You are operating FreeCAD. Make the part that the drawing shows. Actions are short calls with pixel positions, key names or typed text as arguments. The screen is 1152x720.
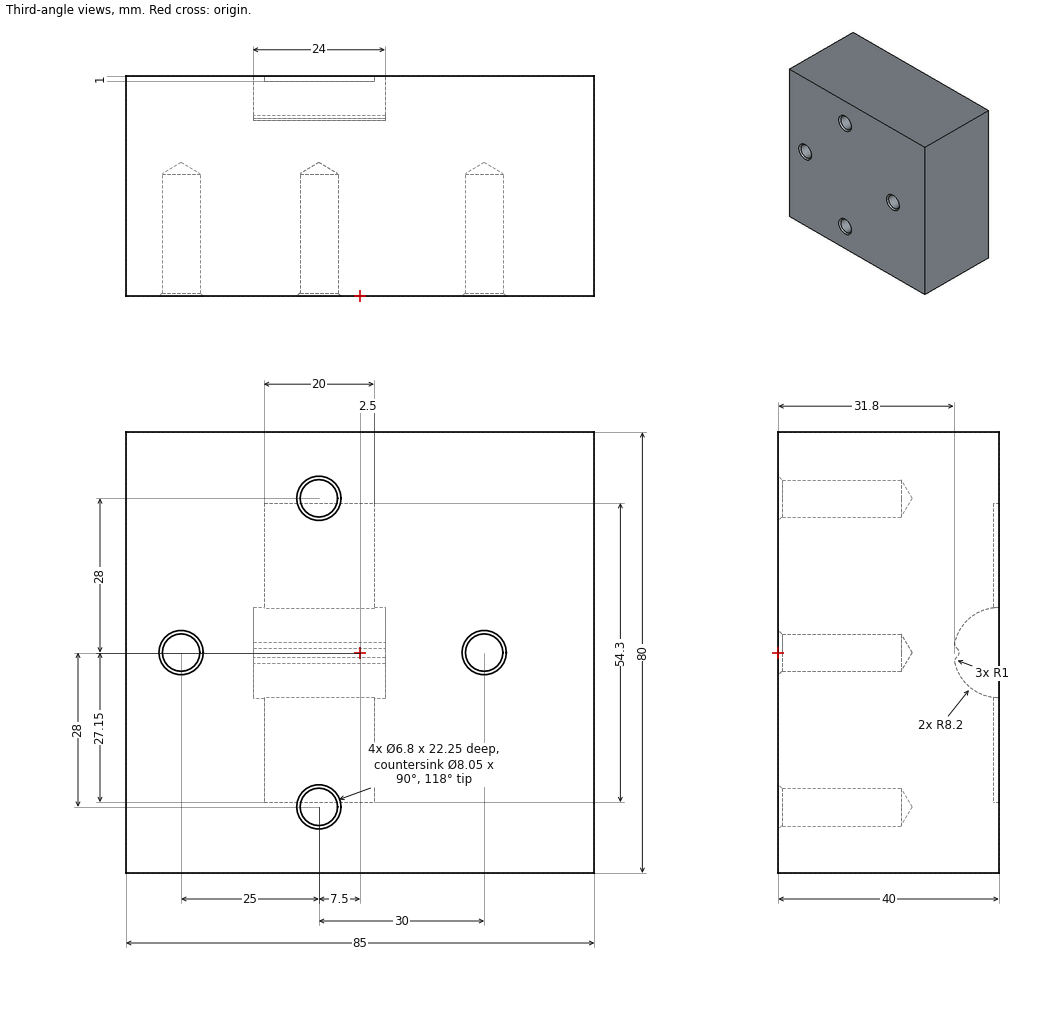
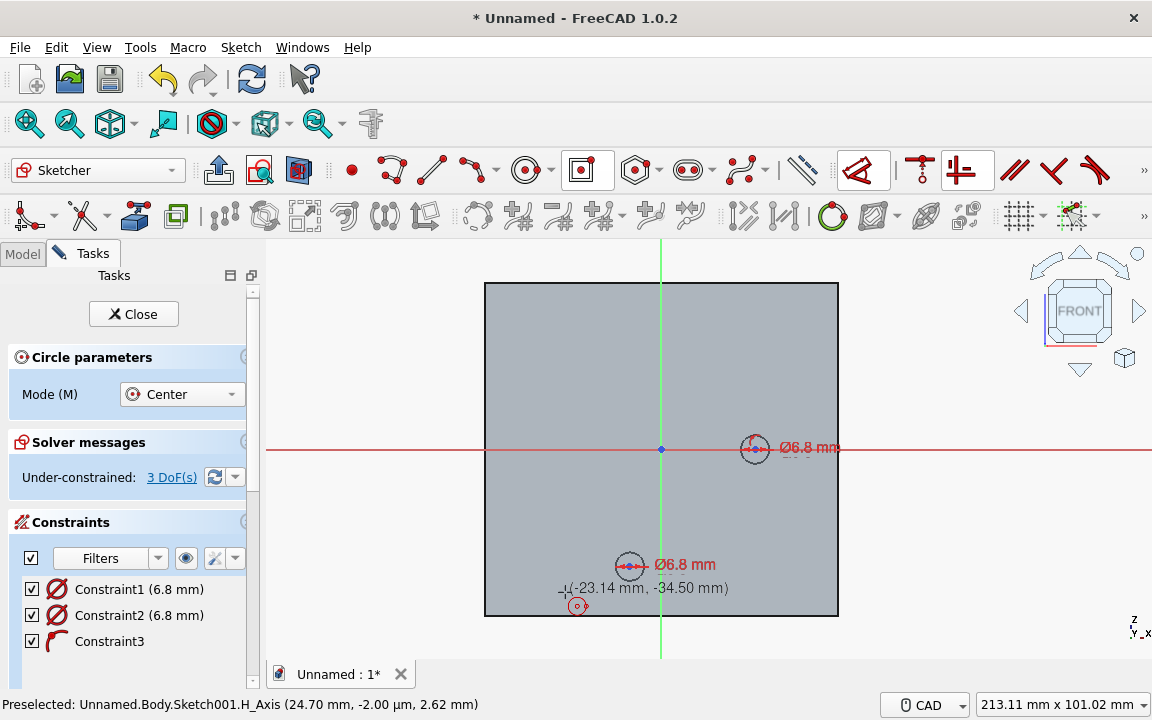
scroll(630, 333, up, 3)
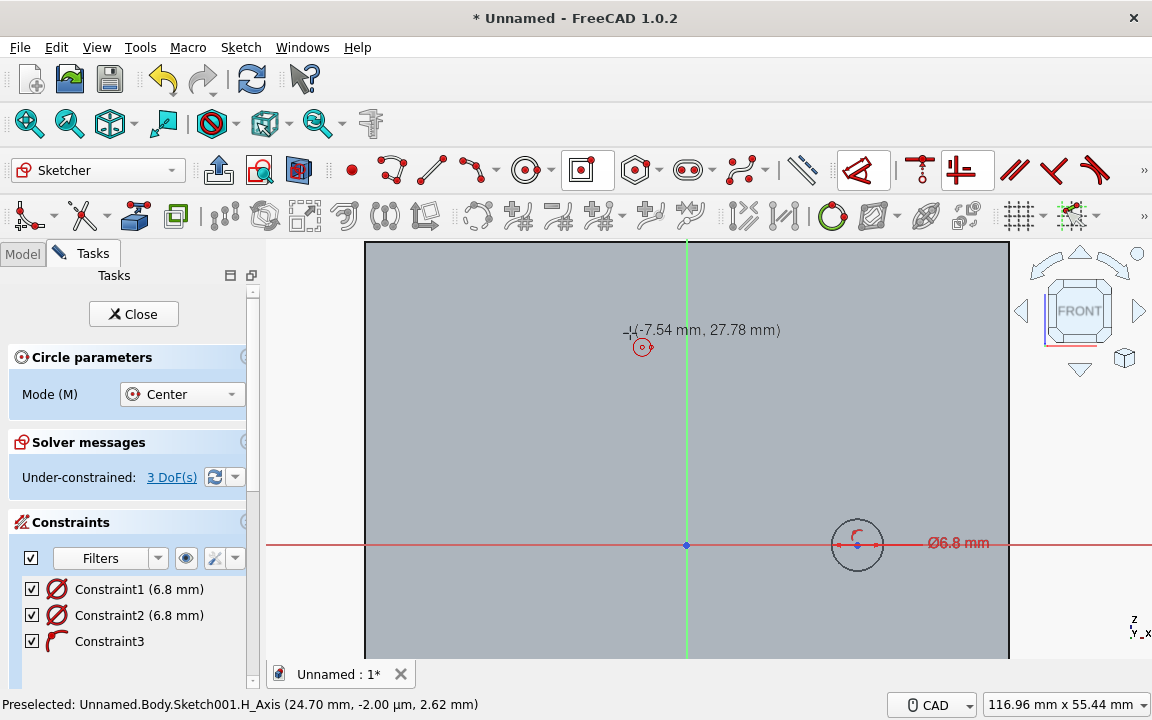
click(630, 333)
move(648, 315)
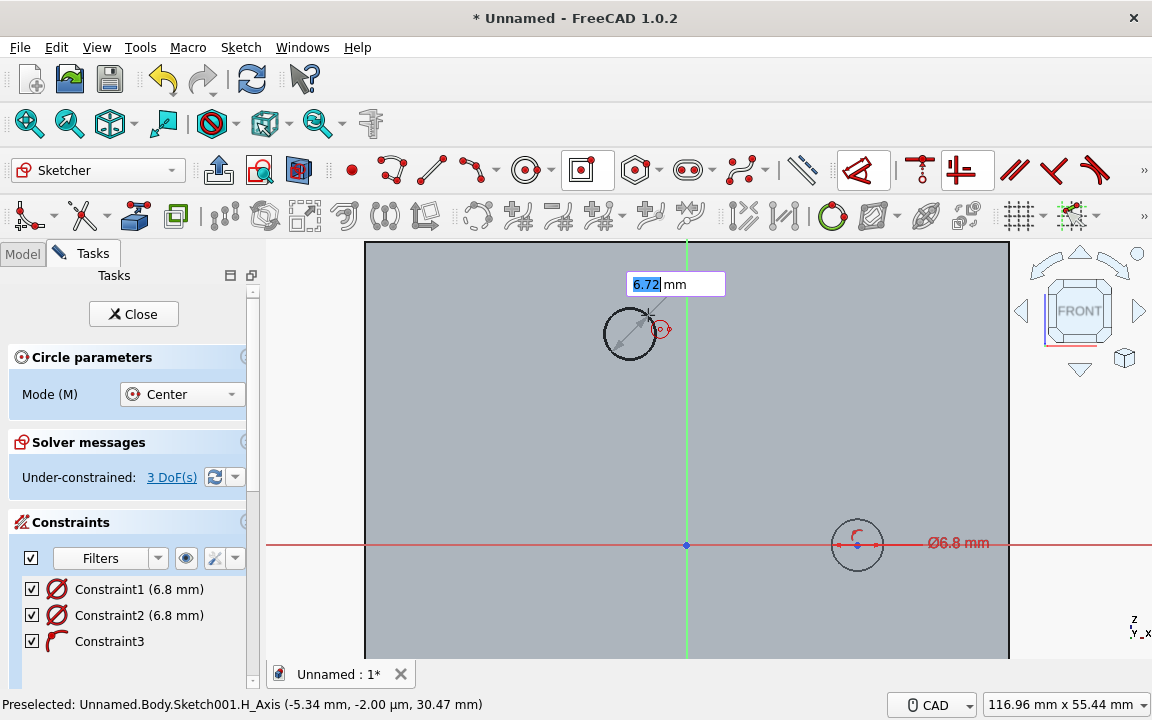
text(6.8)
key(Return)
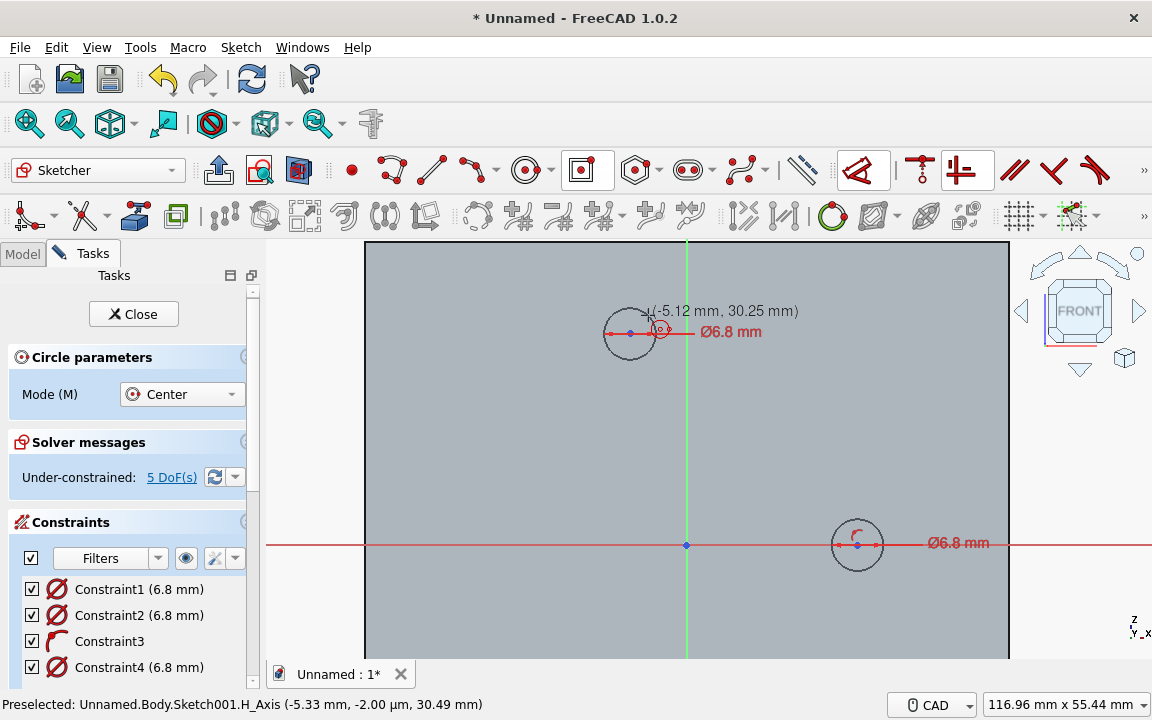
click(441, 545)
move(459, 527)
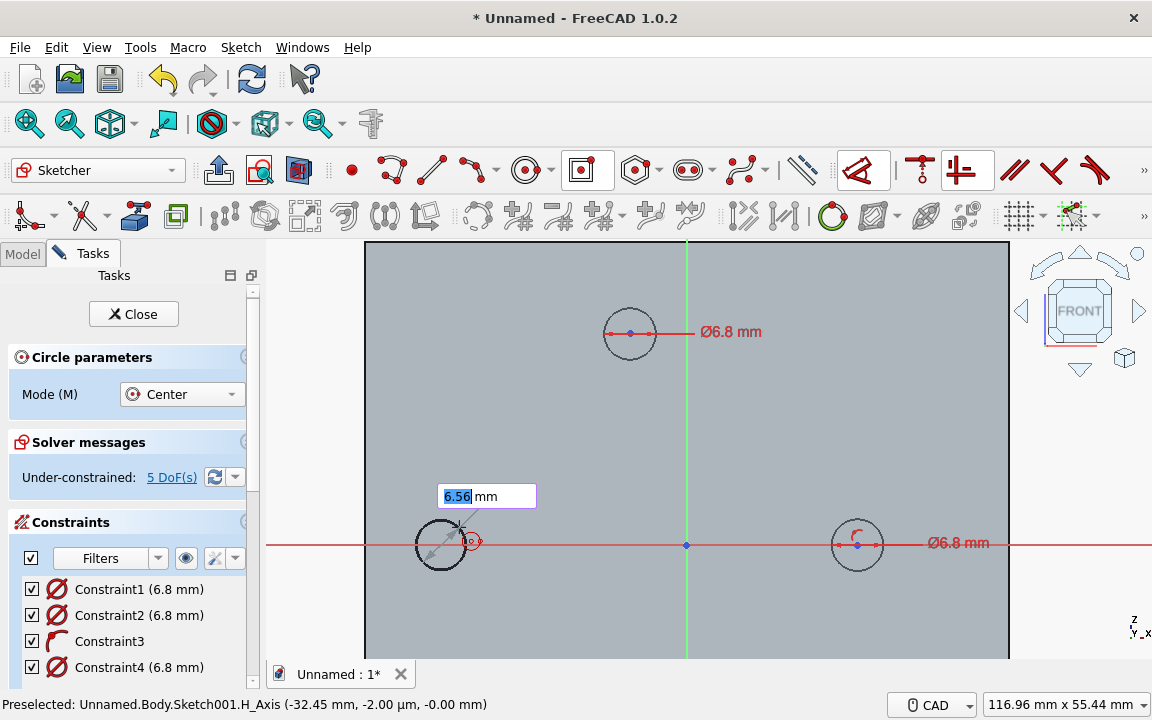
text(6.8)
key(Return)
key(Escape)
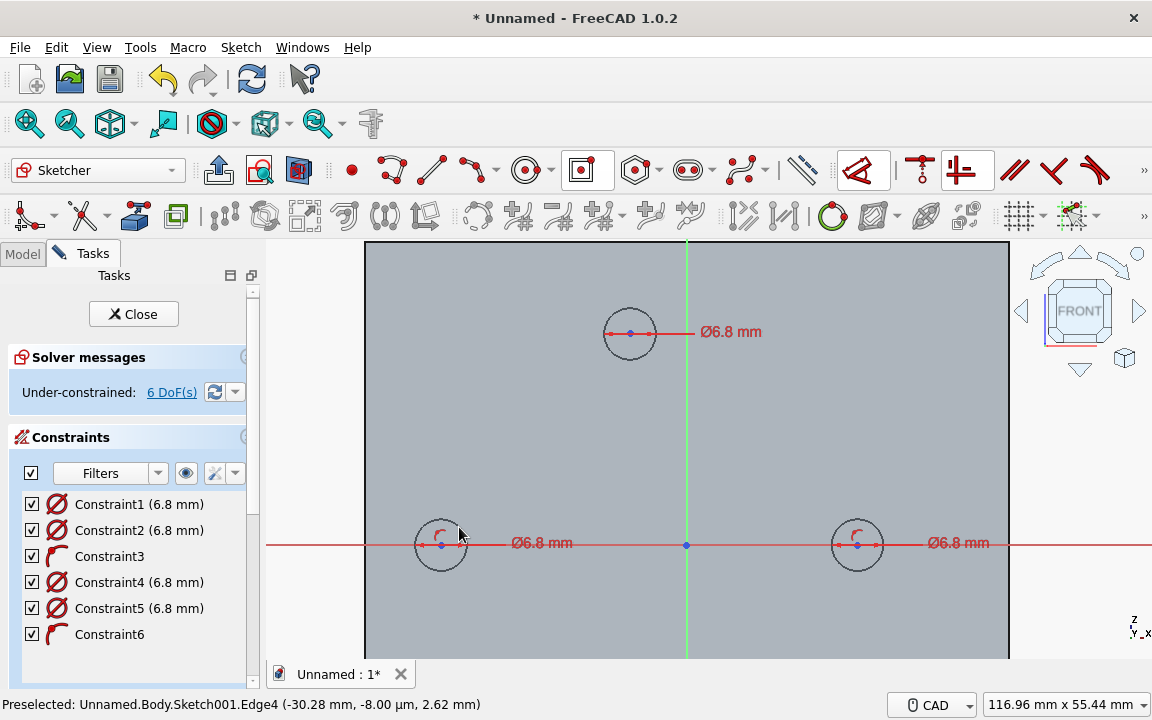
scroll(630, 332, down, 3)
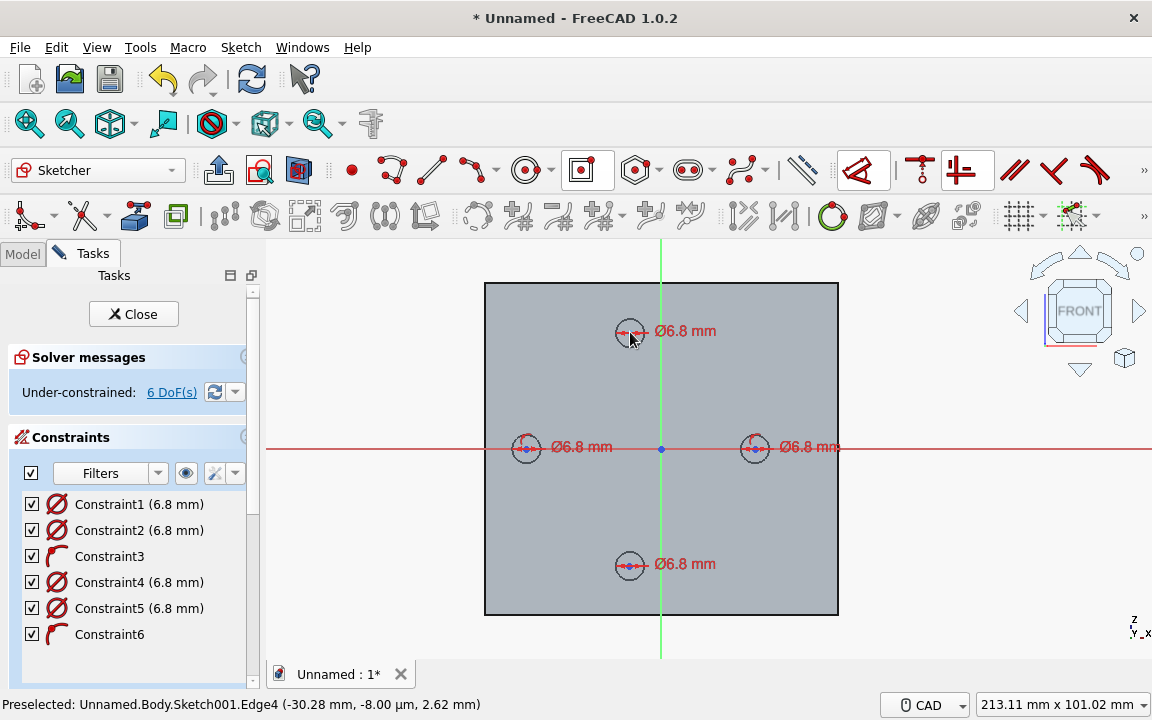
click(630, 566)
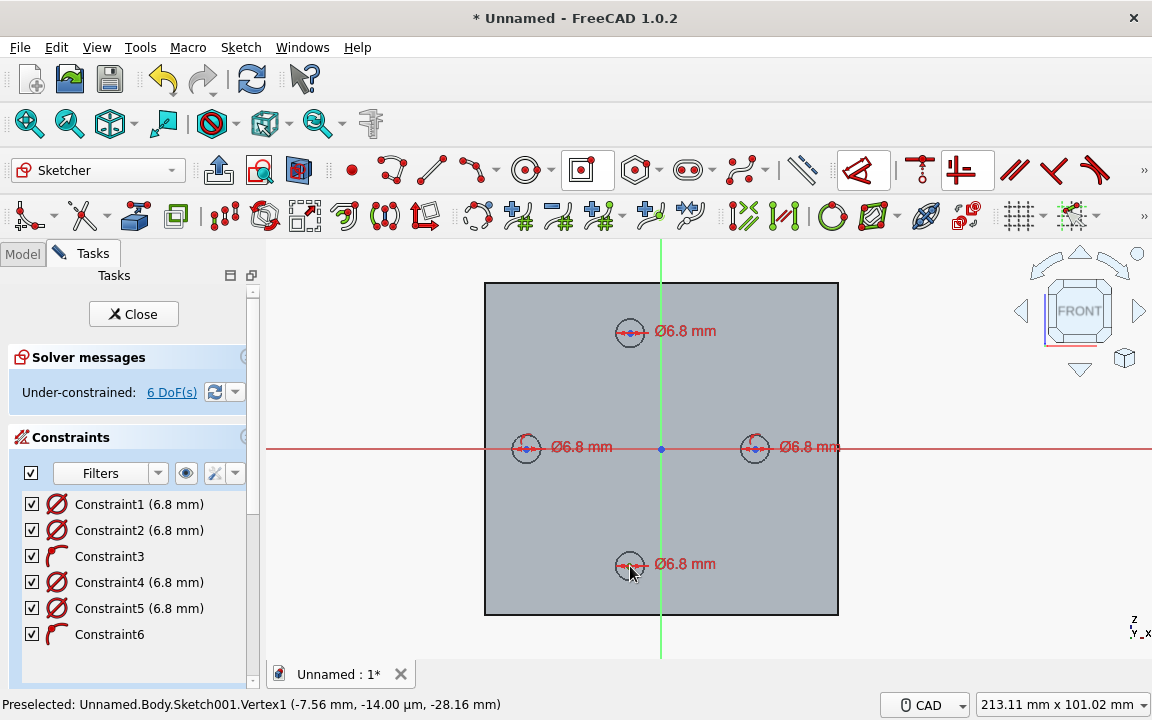
click(630, 333)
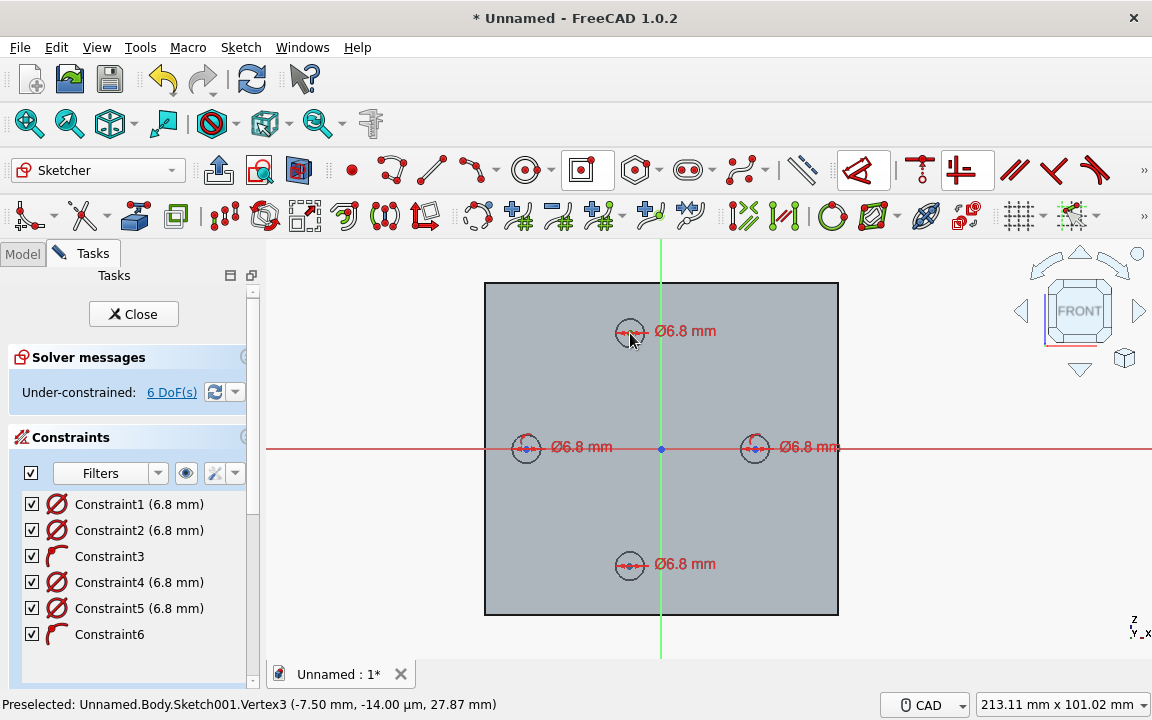
key(v)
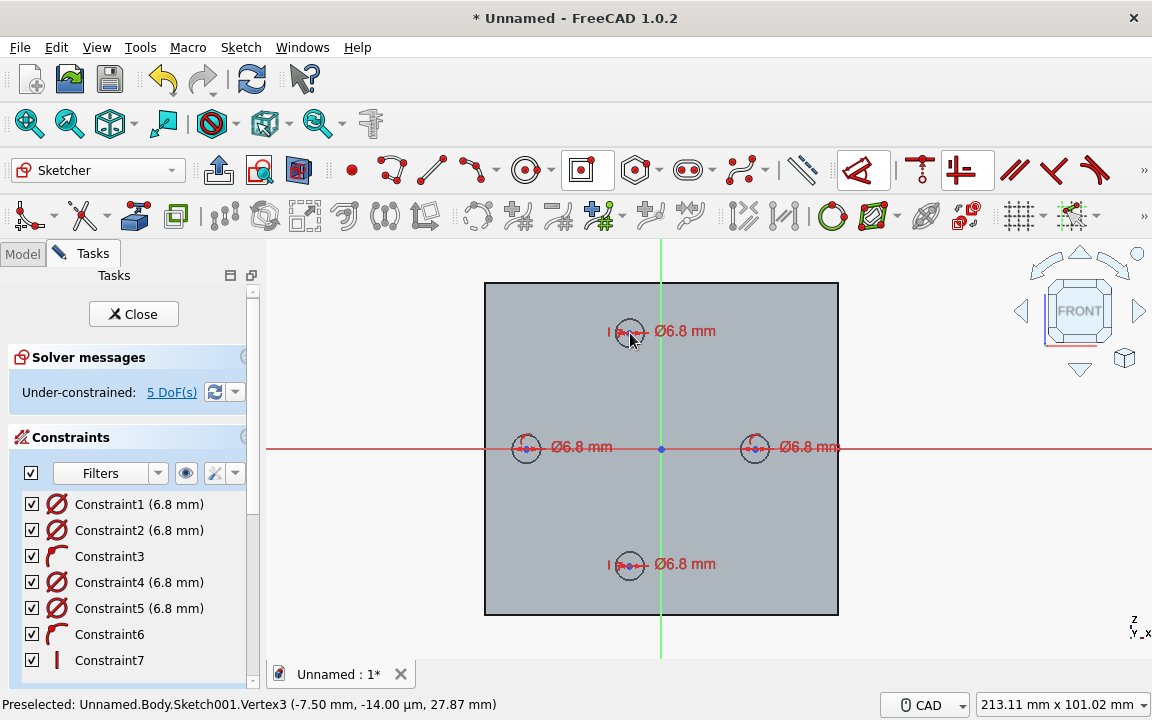
click(858, 170)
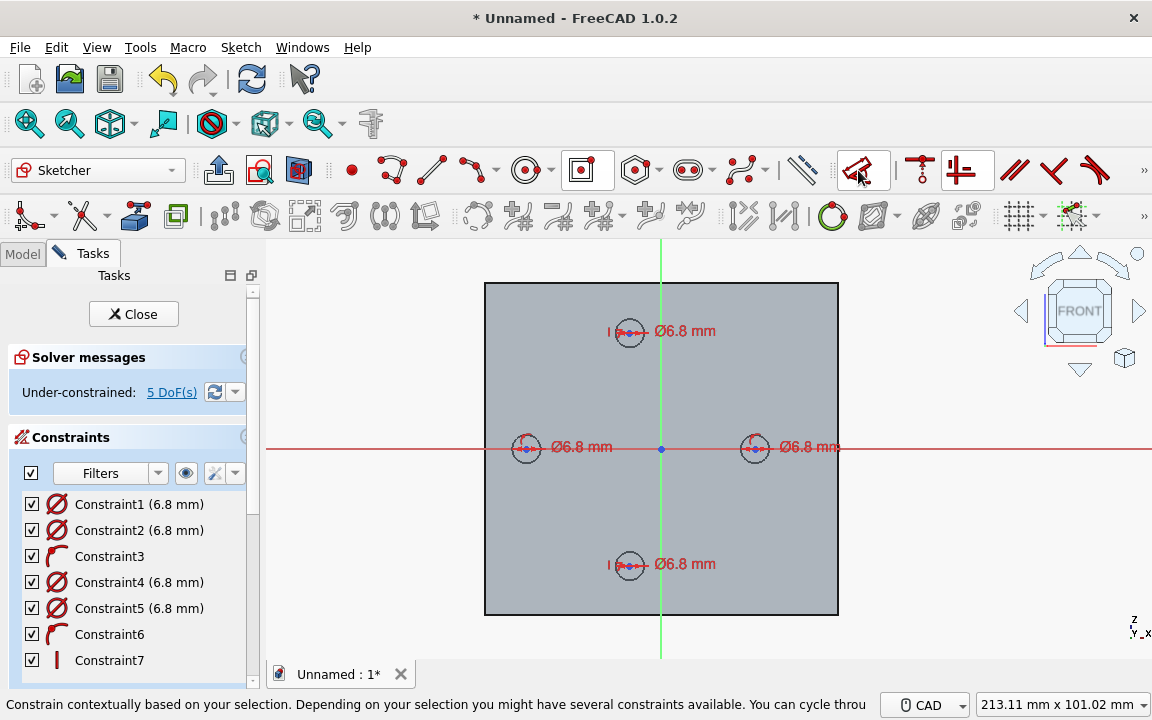
click(630, 566)
click(695, 508)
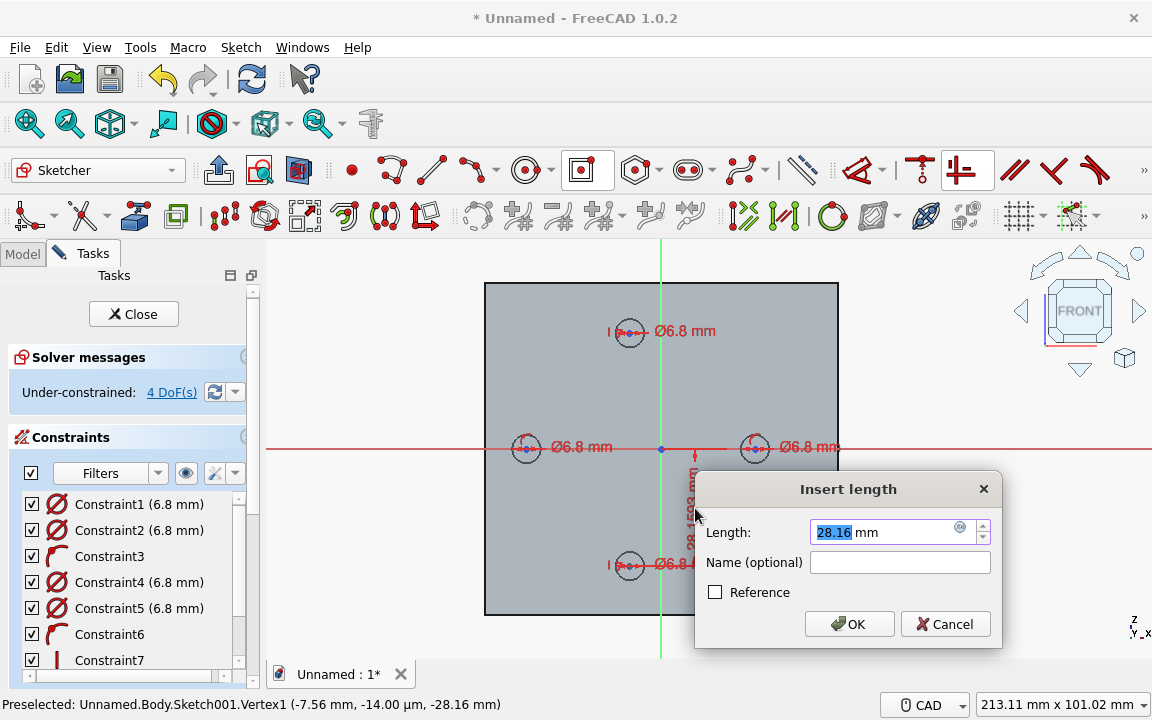
text(28)
key(Return)